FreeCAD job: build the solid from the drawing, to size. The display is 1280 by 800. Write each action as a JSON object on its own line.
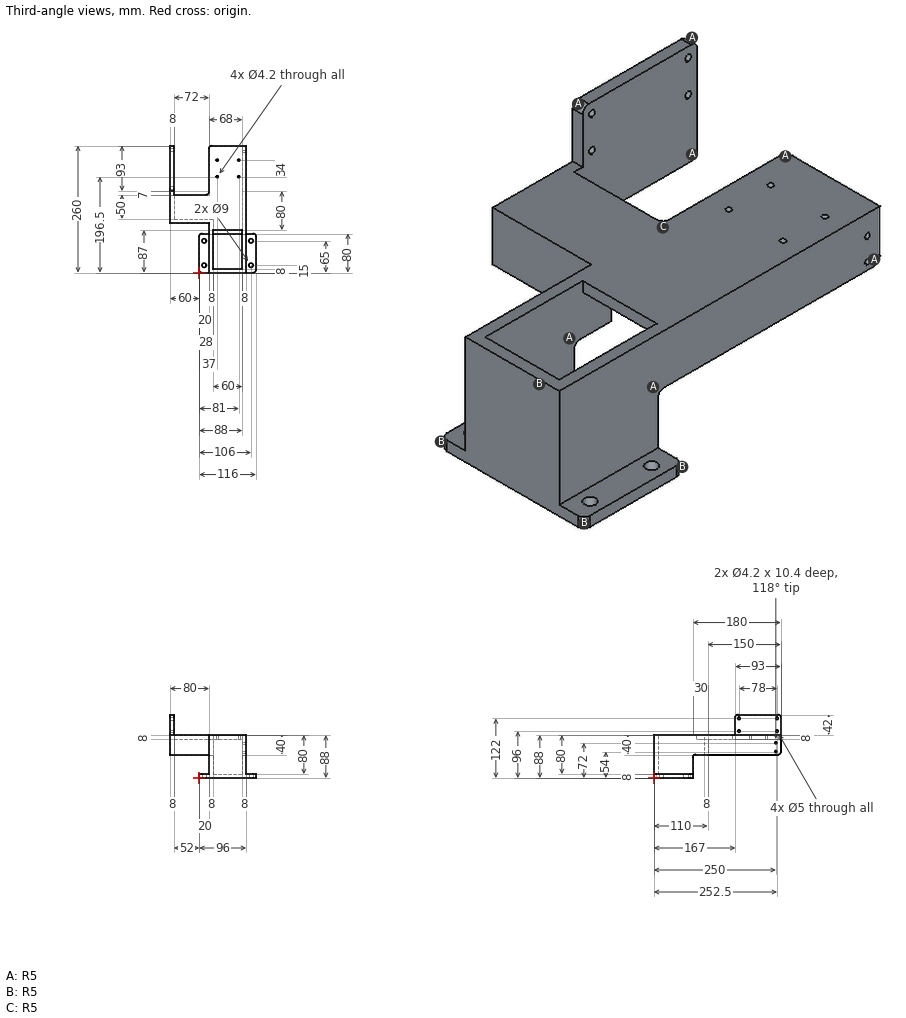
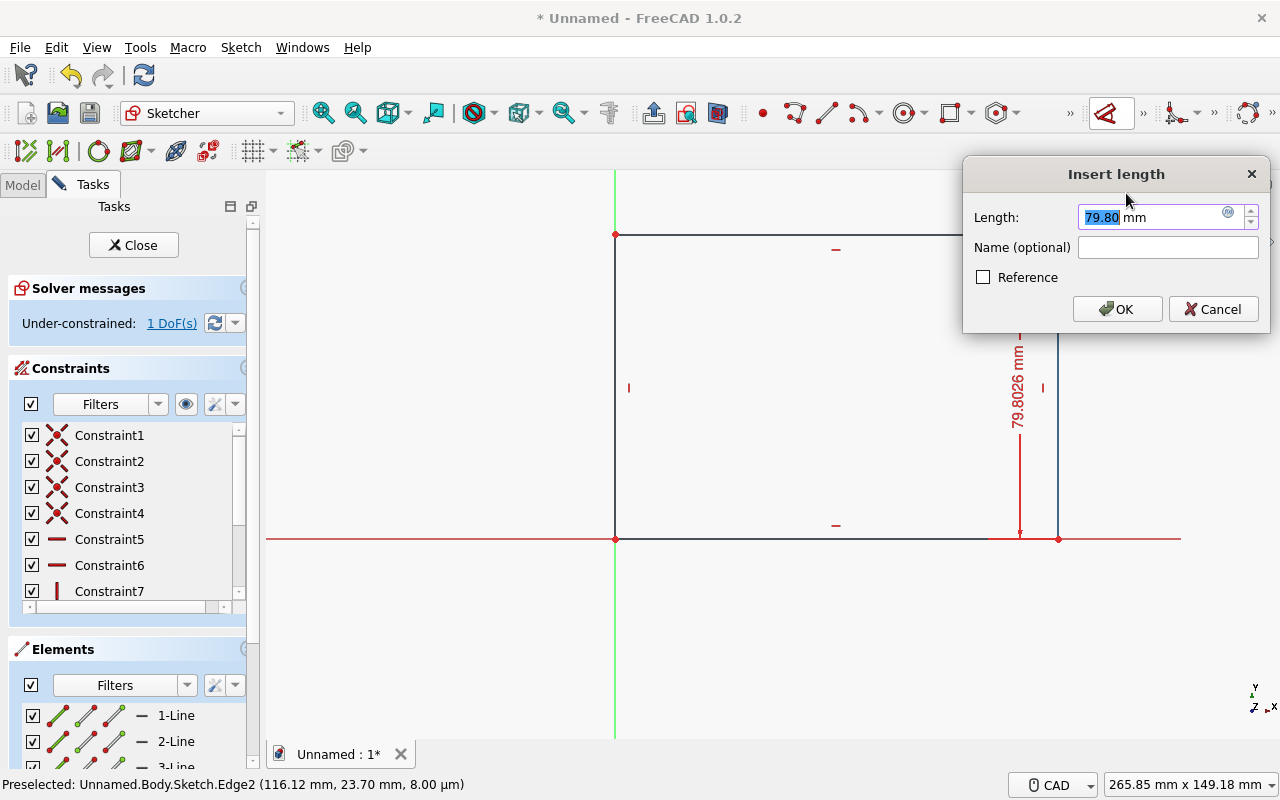
{"action": "type", "text": "80"}
{"action": "key", "text": "Return"}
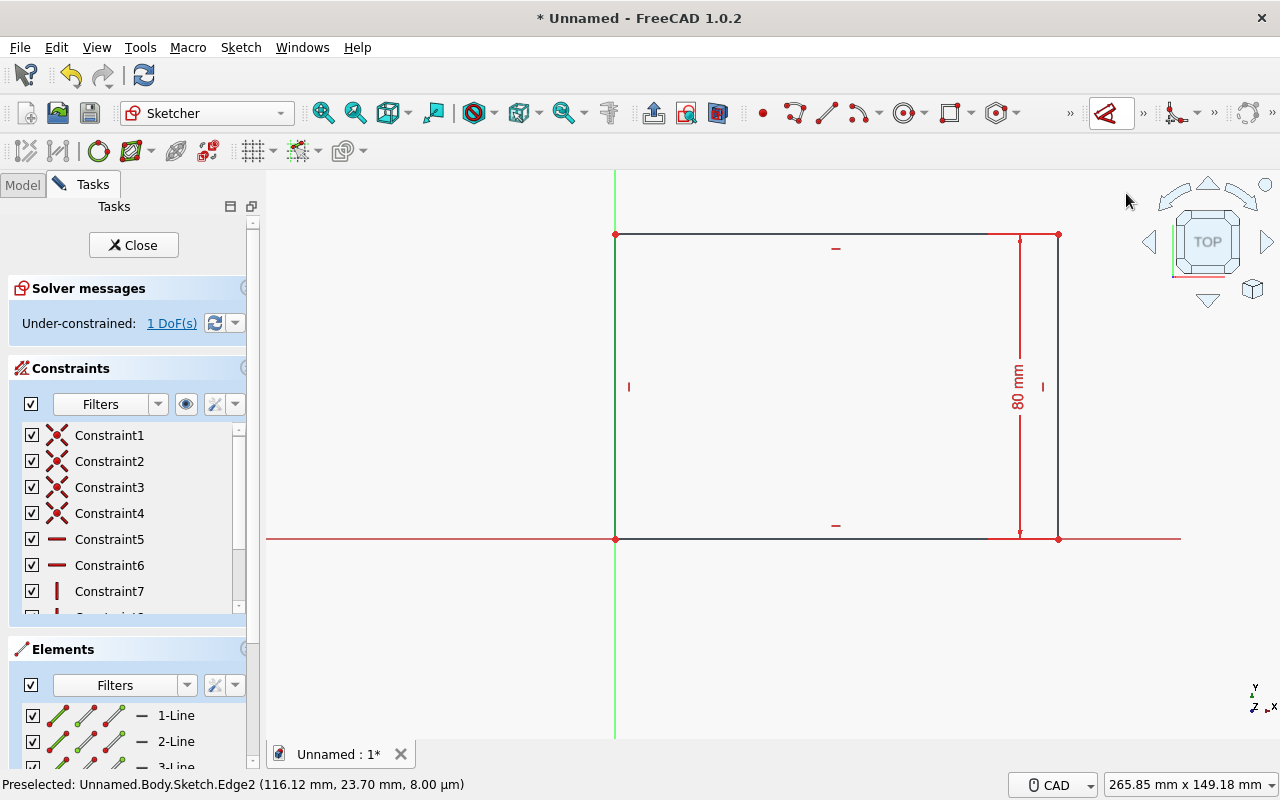
{"action": "left_click", "coordinate": [748, 539]}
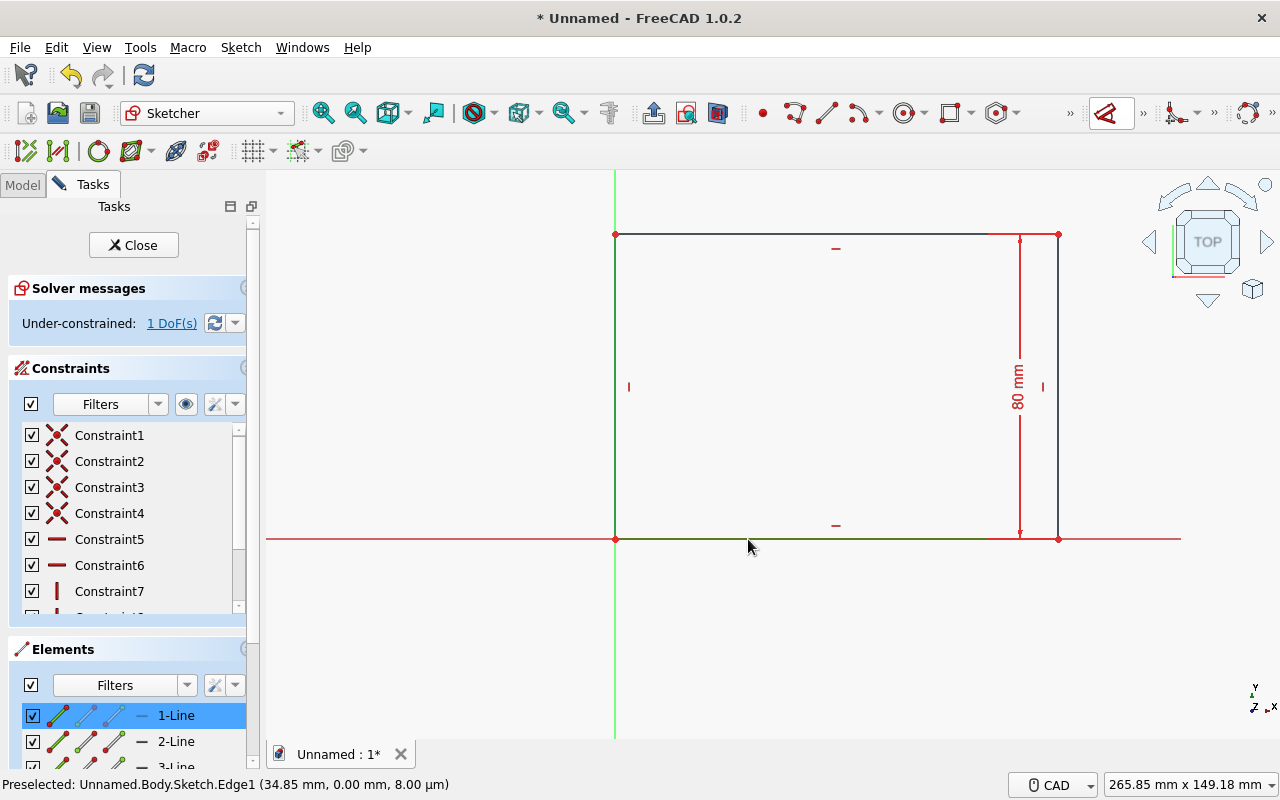
{"action": "key", "text": "l"}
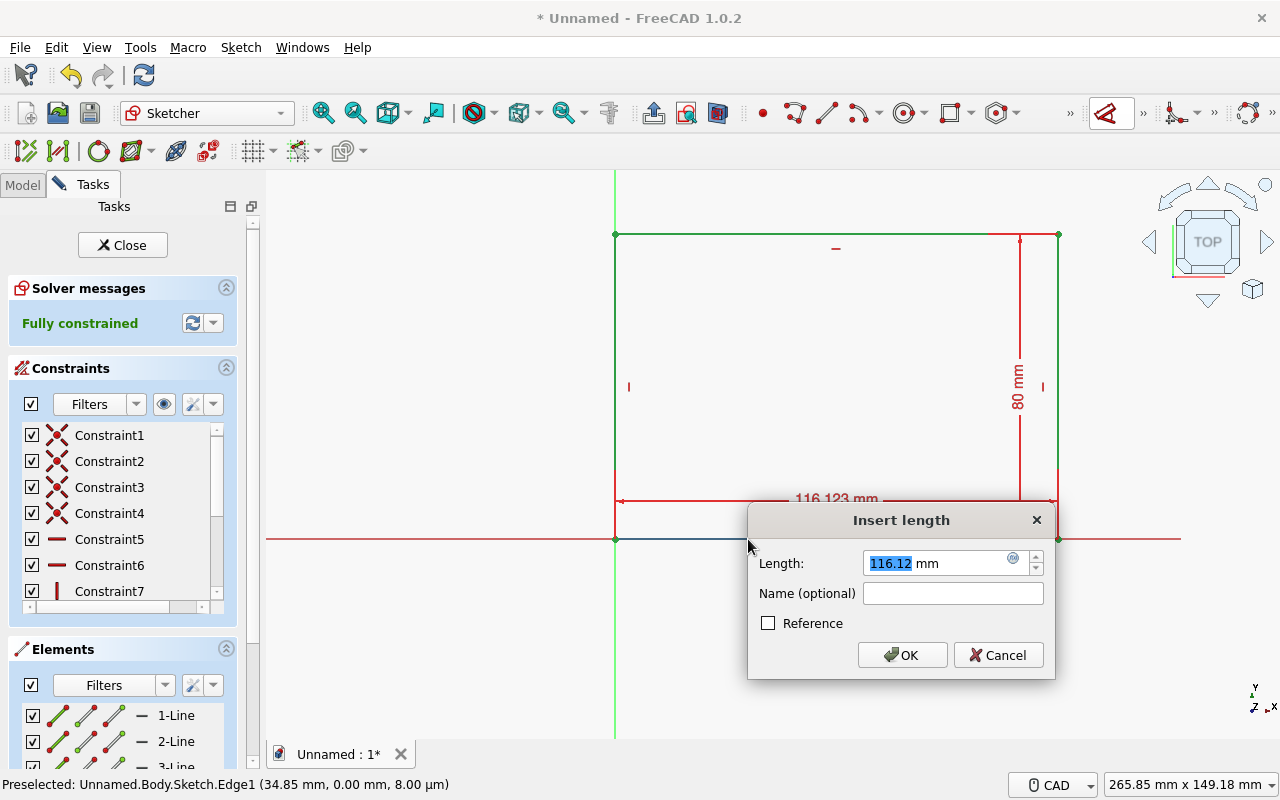
{"action": "type", "text": "116"}
{"action": "key", "text": "Return"}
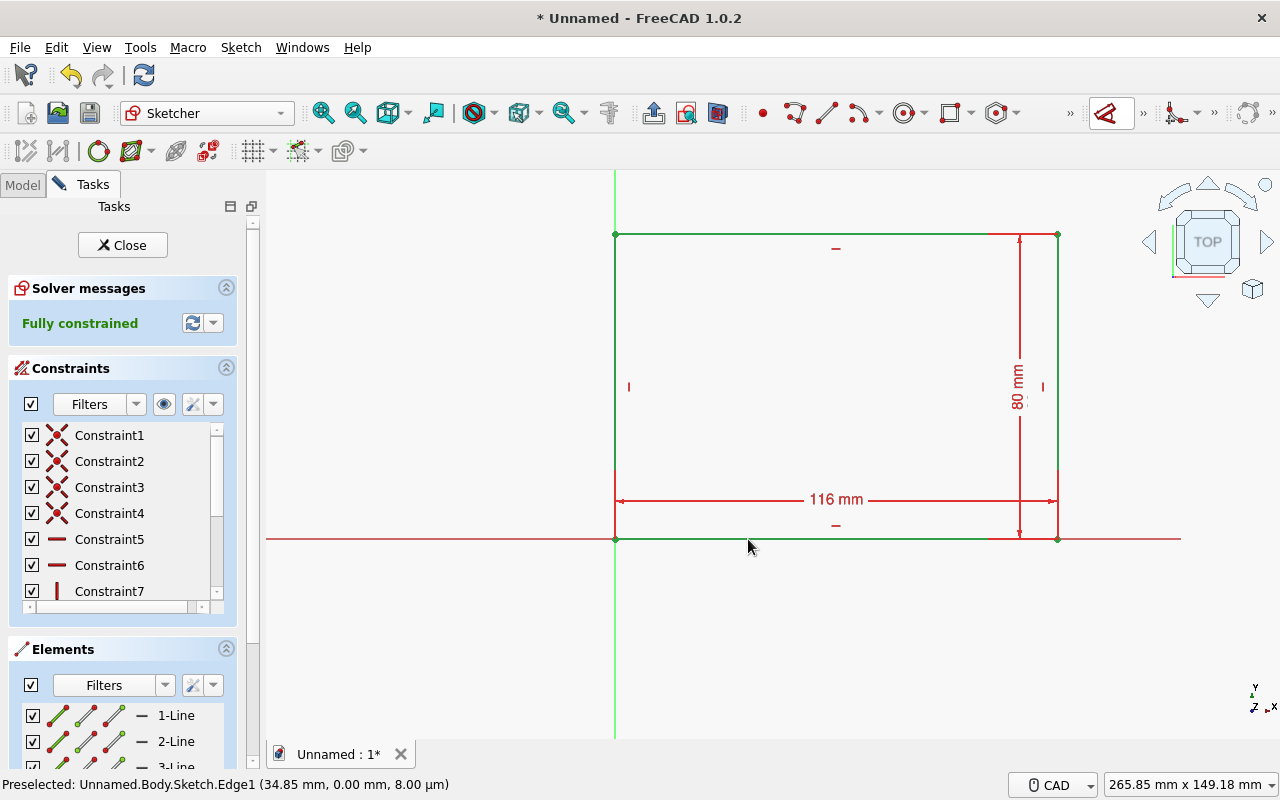
{"action": "left_click", "coordinate": [123, 245]}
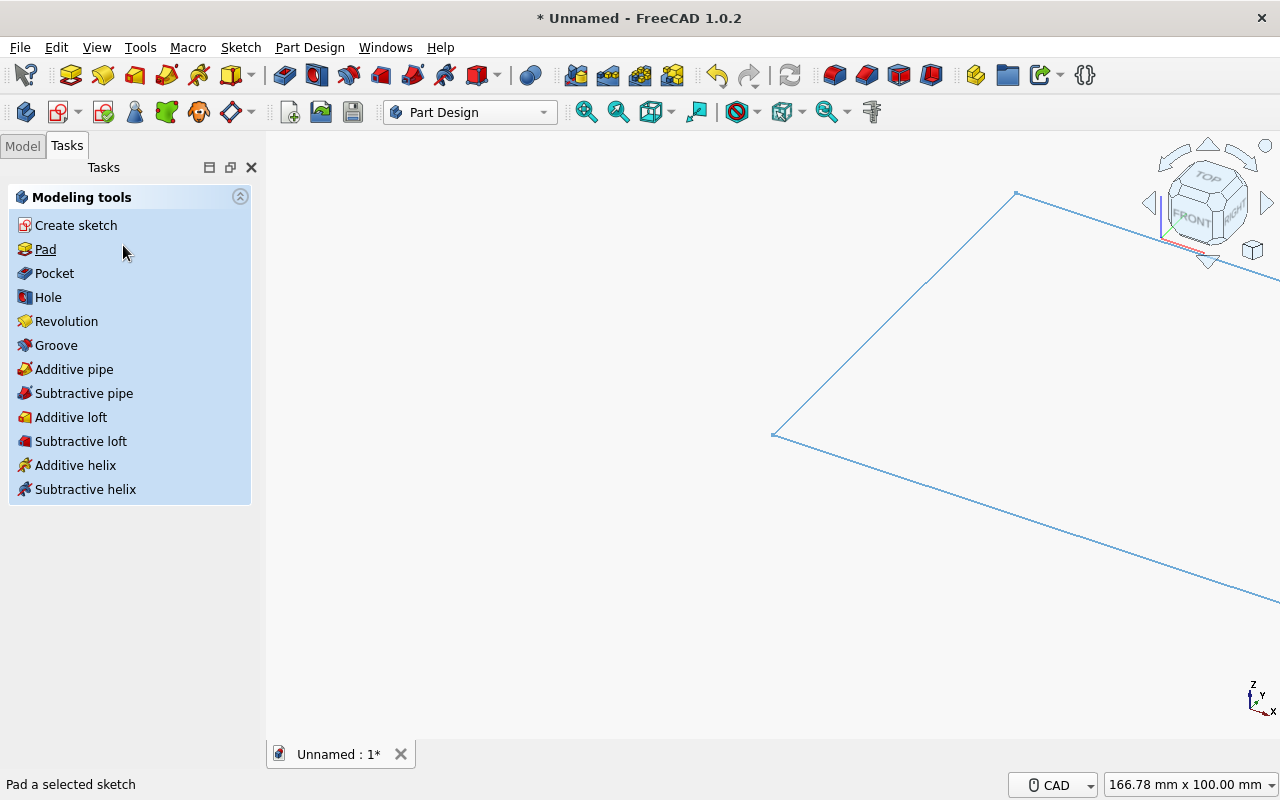
{"action": "left_click", "coordinate": [72, 76]}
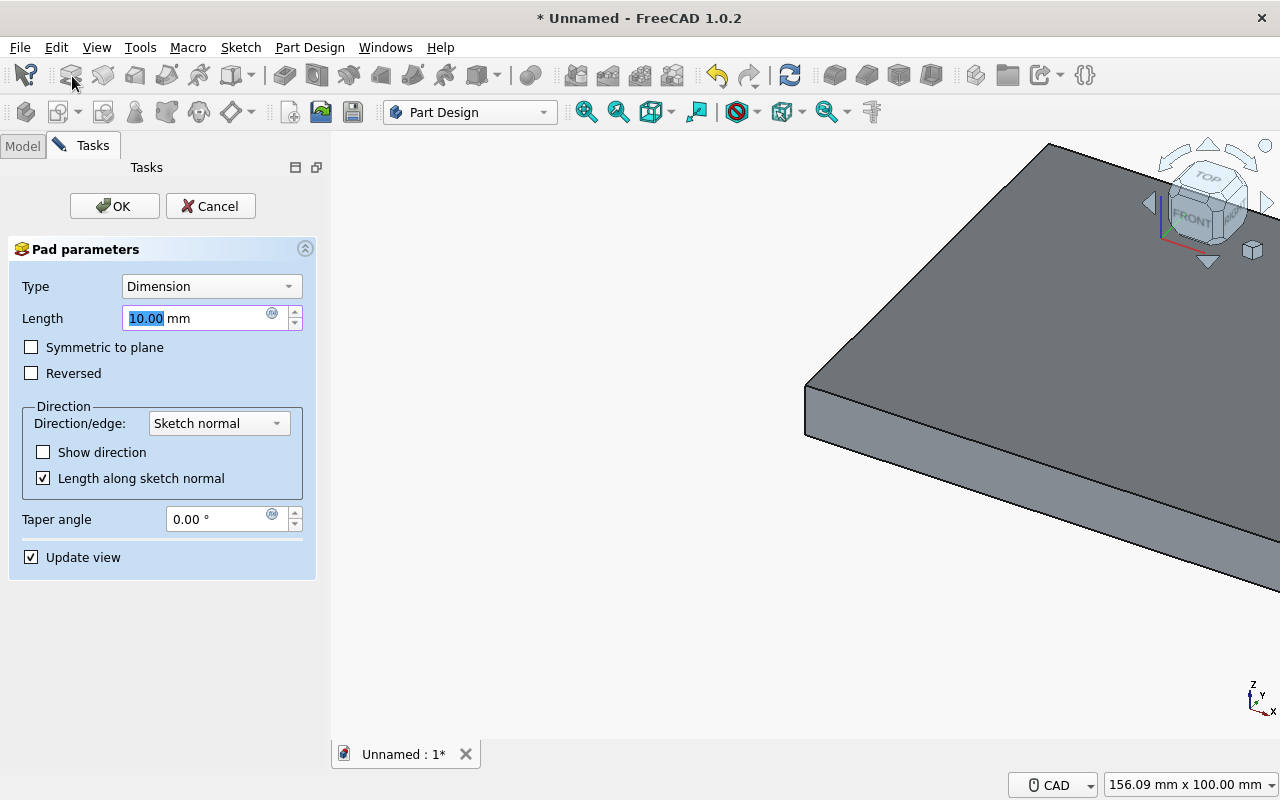
{"action": "type", "text": "8"}
{"action": "key", "text": "Tab"}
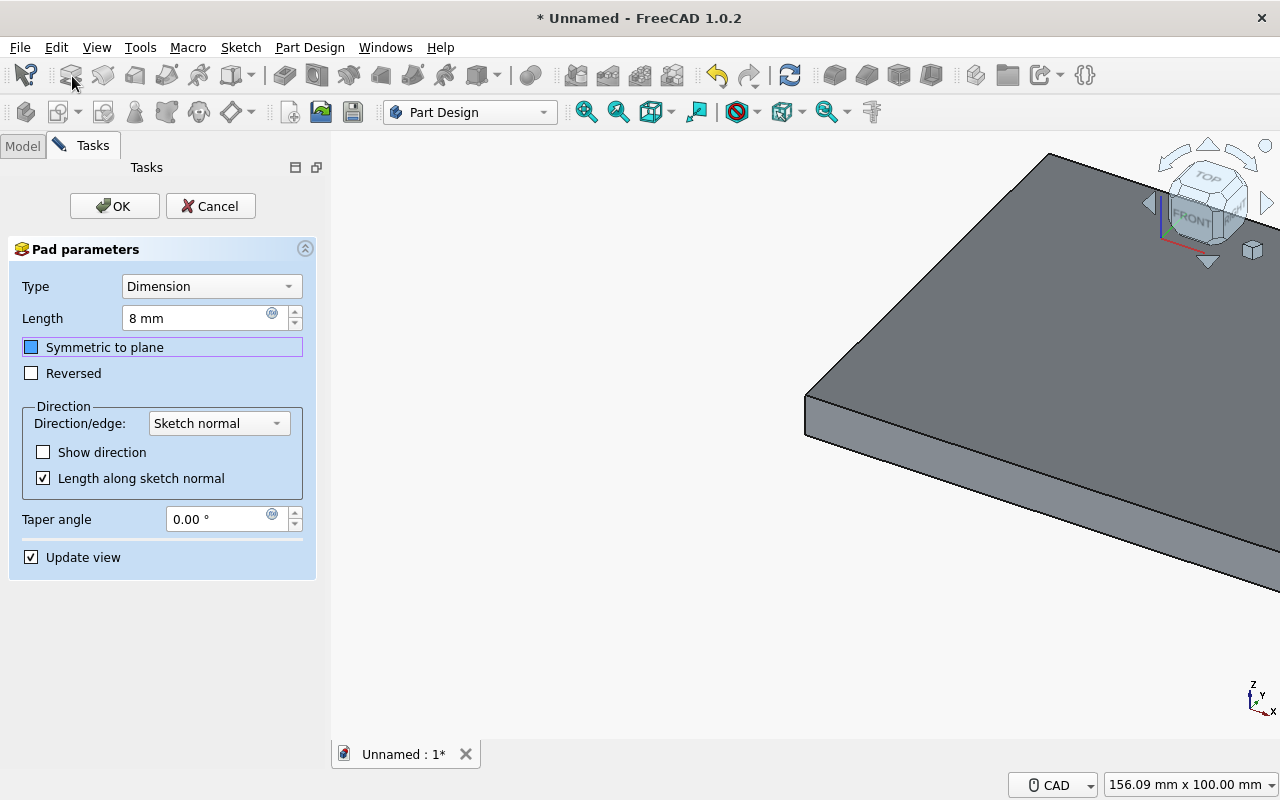
{"action": "left_click", "coordinate": [115, 206]}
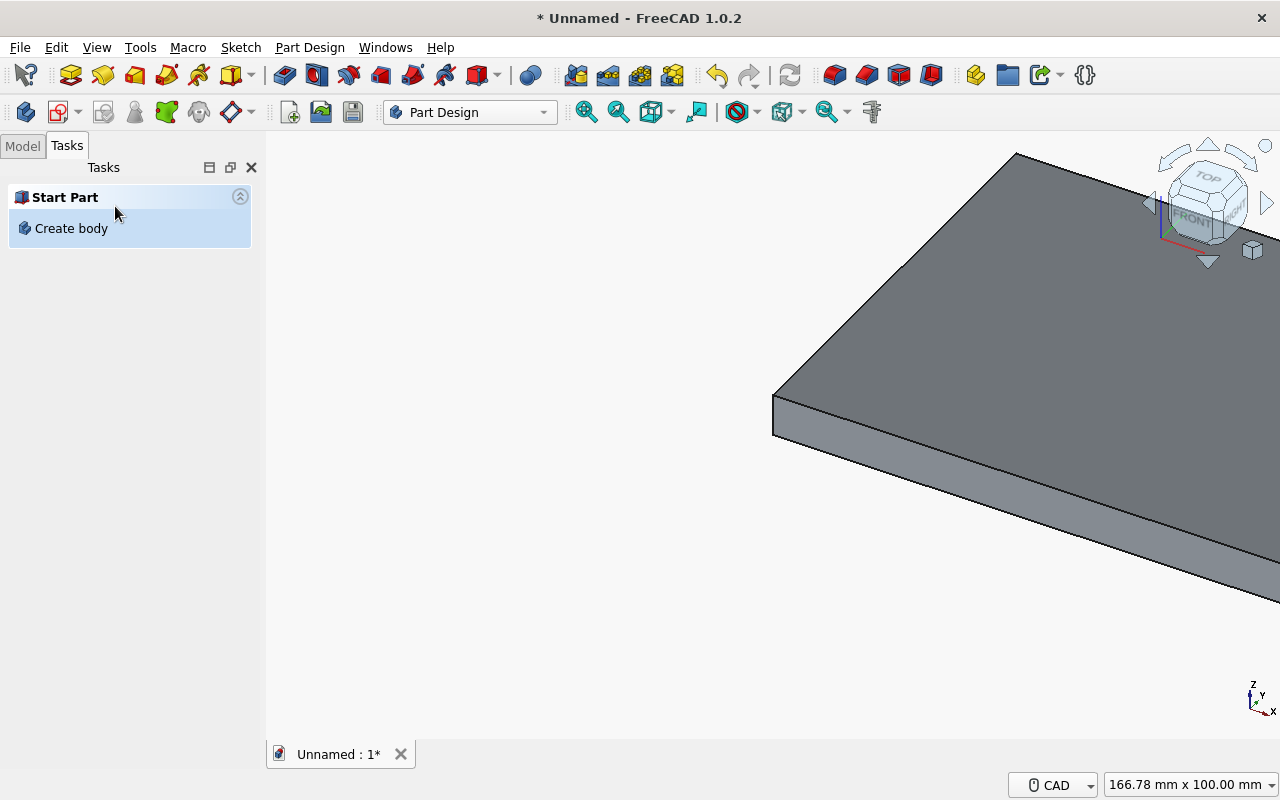
{"action": "left_click", "coordinate": [588, 112]}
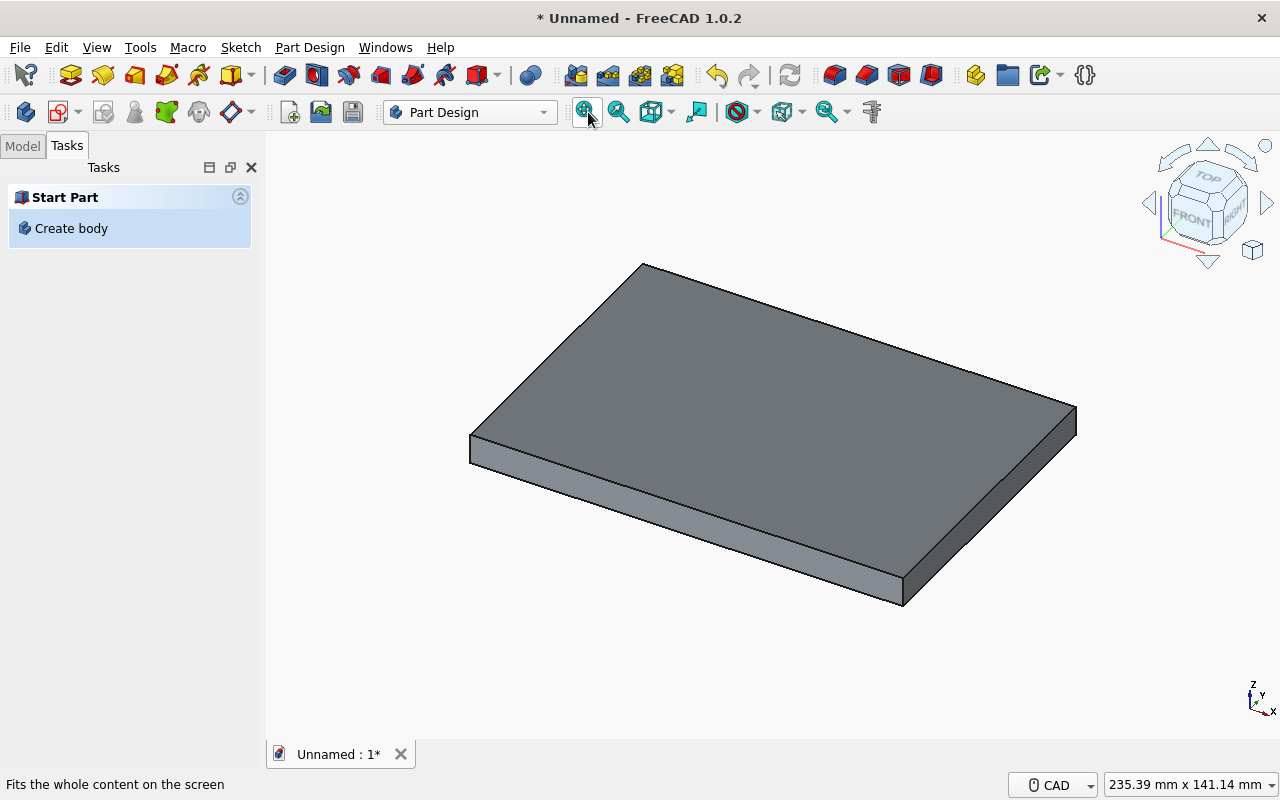
{"action": "left_click", "coordinate": [835, 440]}